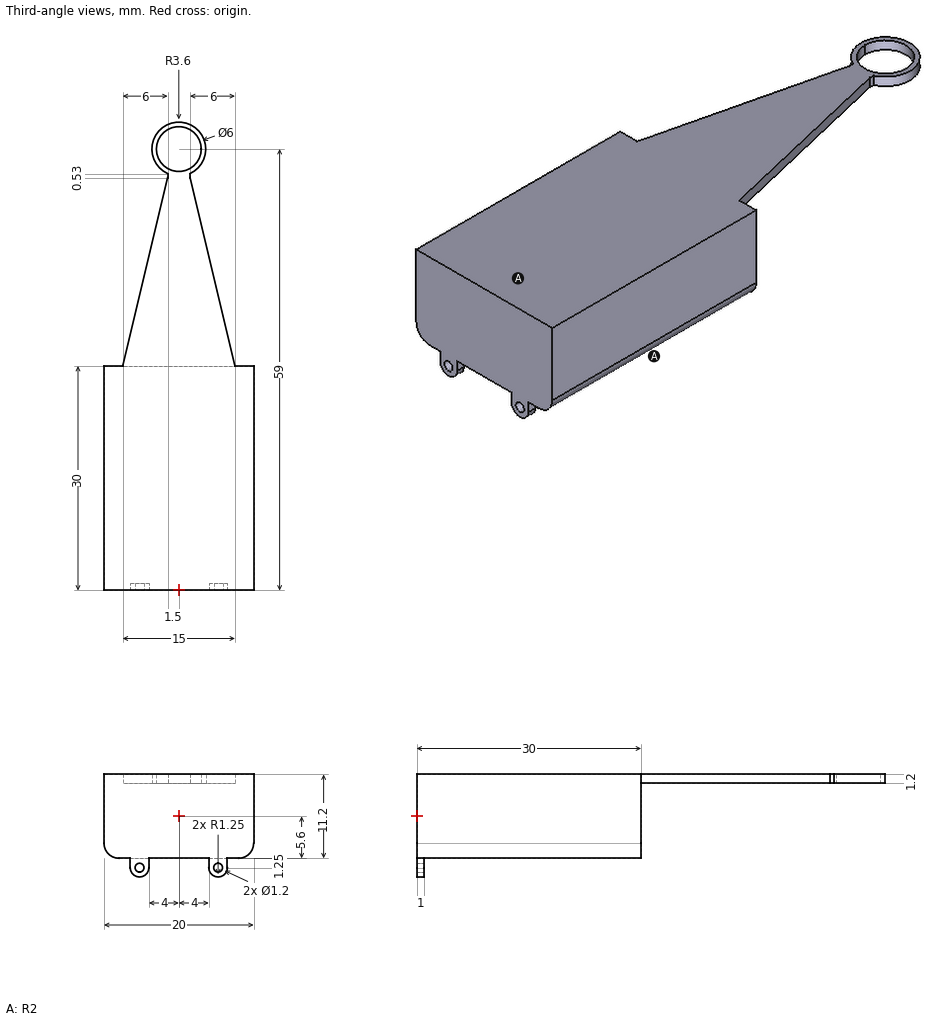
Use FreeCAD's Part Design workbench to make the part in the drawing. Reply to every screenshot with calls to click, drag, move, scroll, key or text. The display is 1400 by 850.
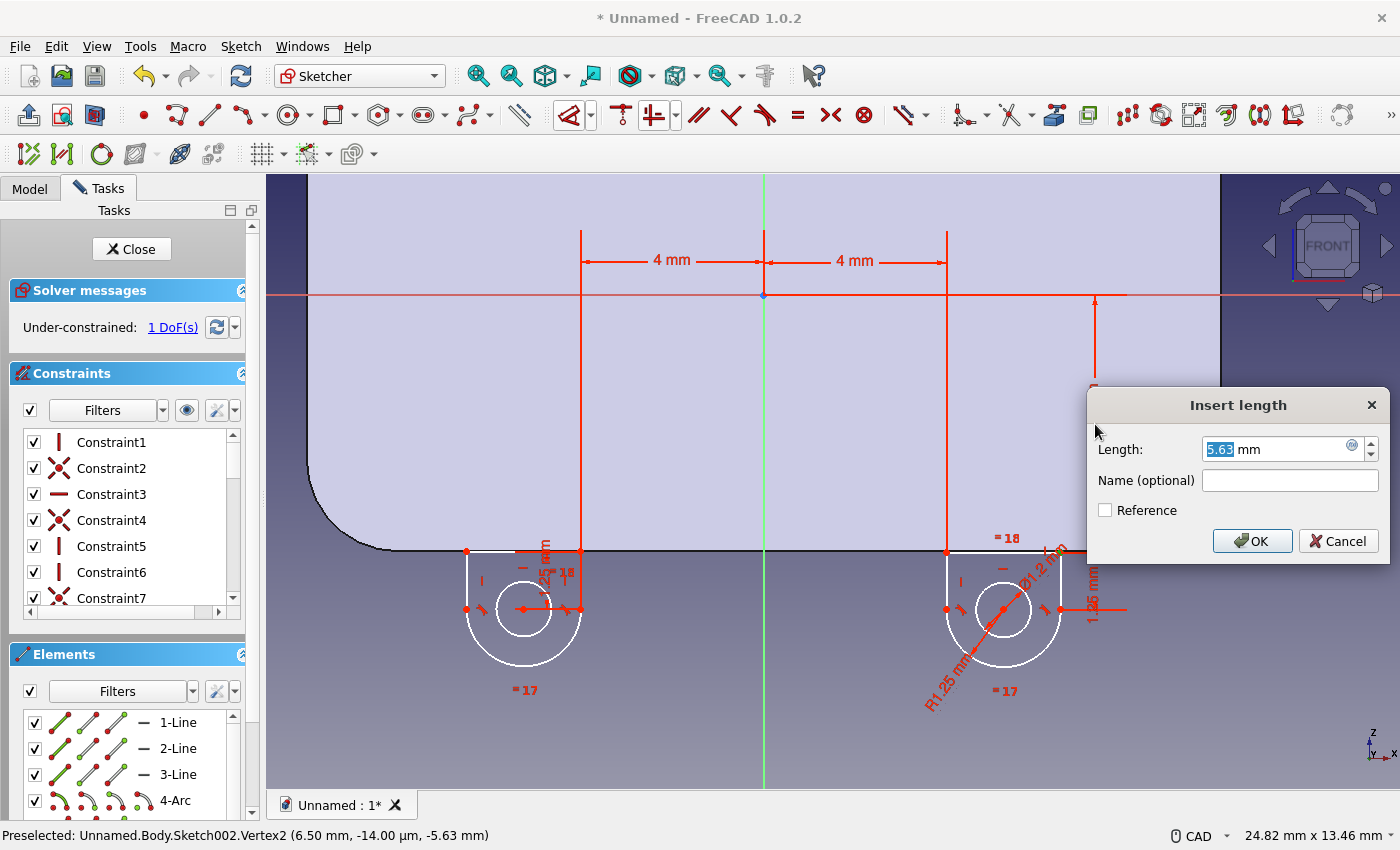
text(5.6)
key(Return)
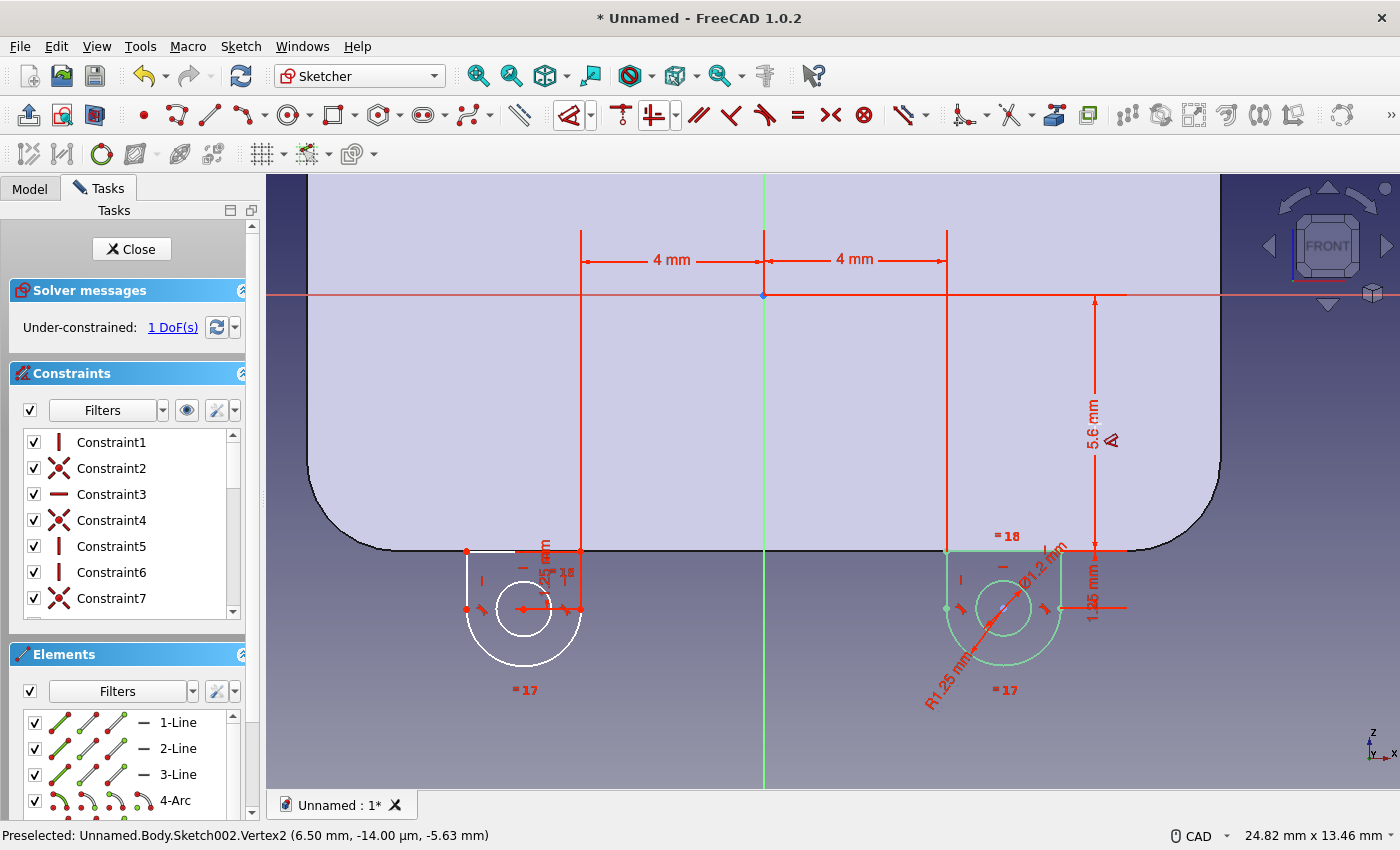
click(581, 552)
click(547, 424)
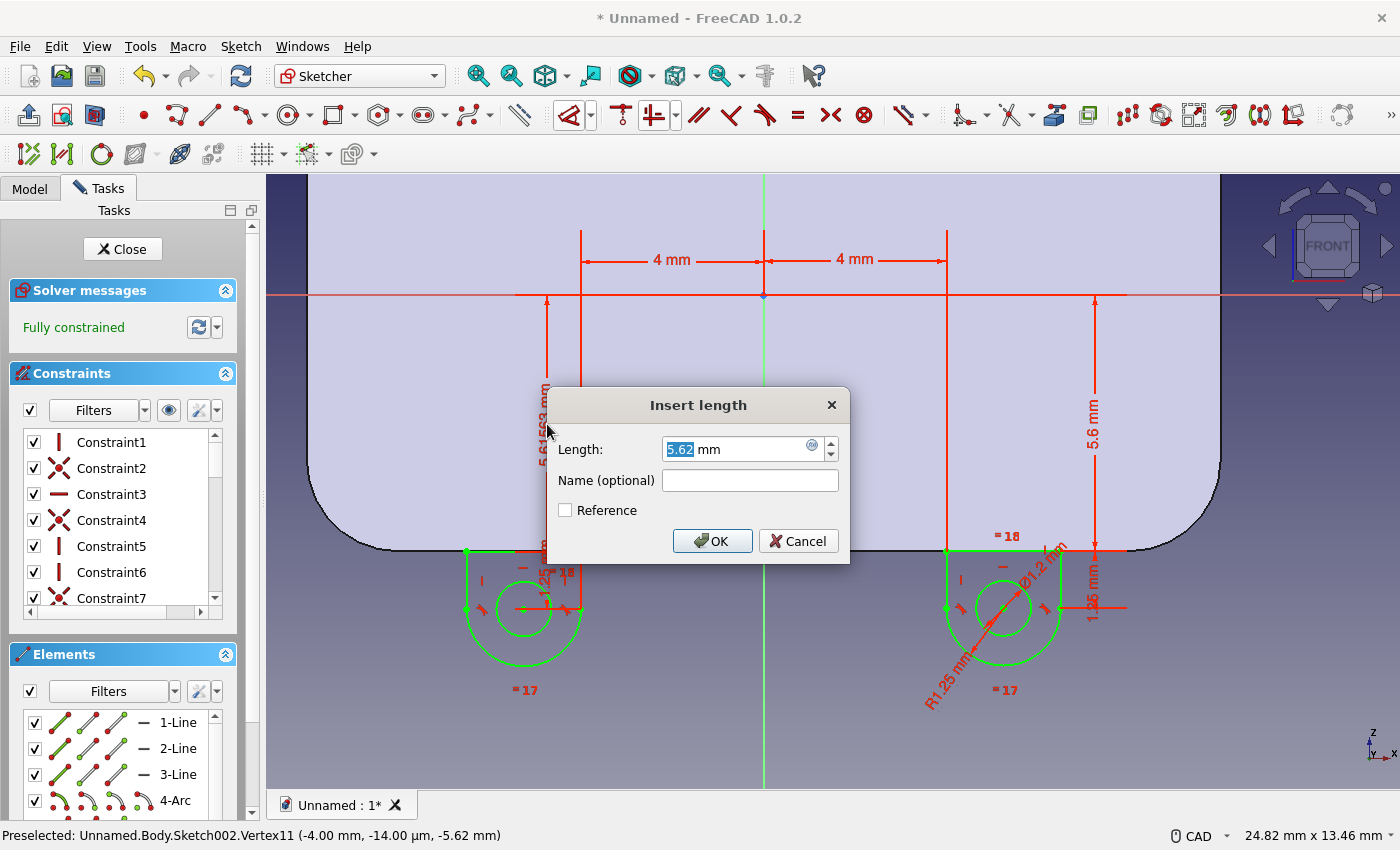
text(5.6)
key(Return)
key(Escape)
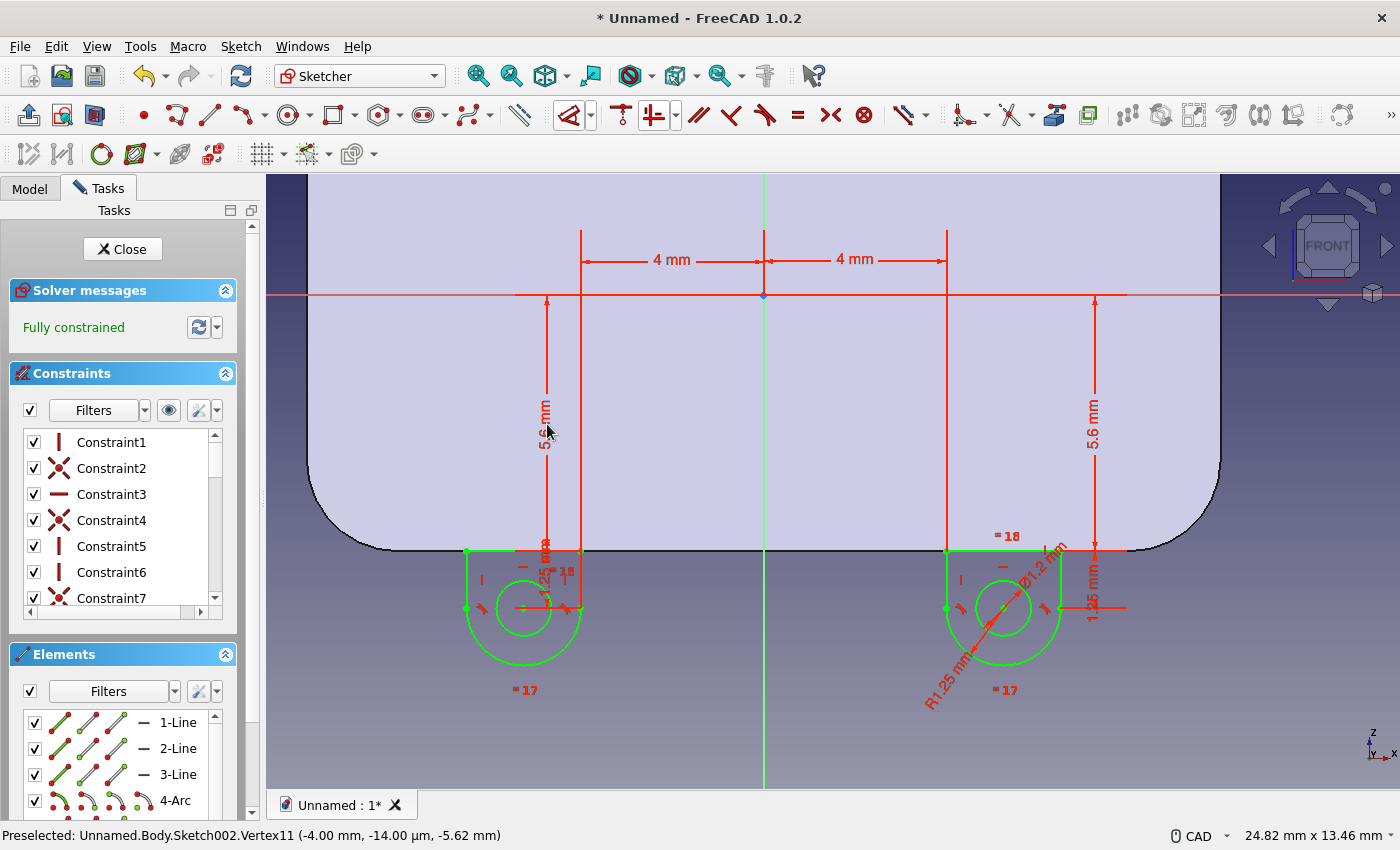
click(123, 249)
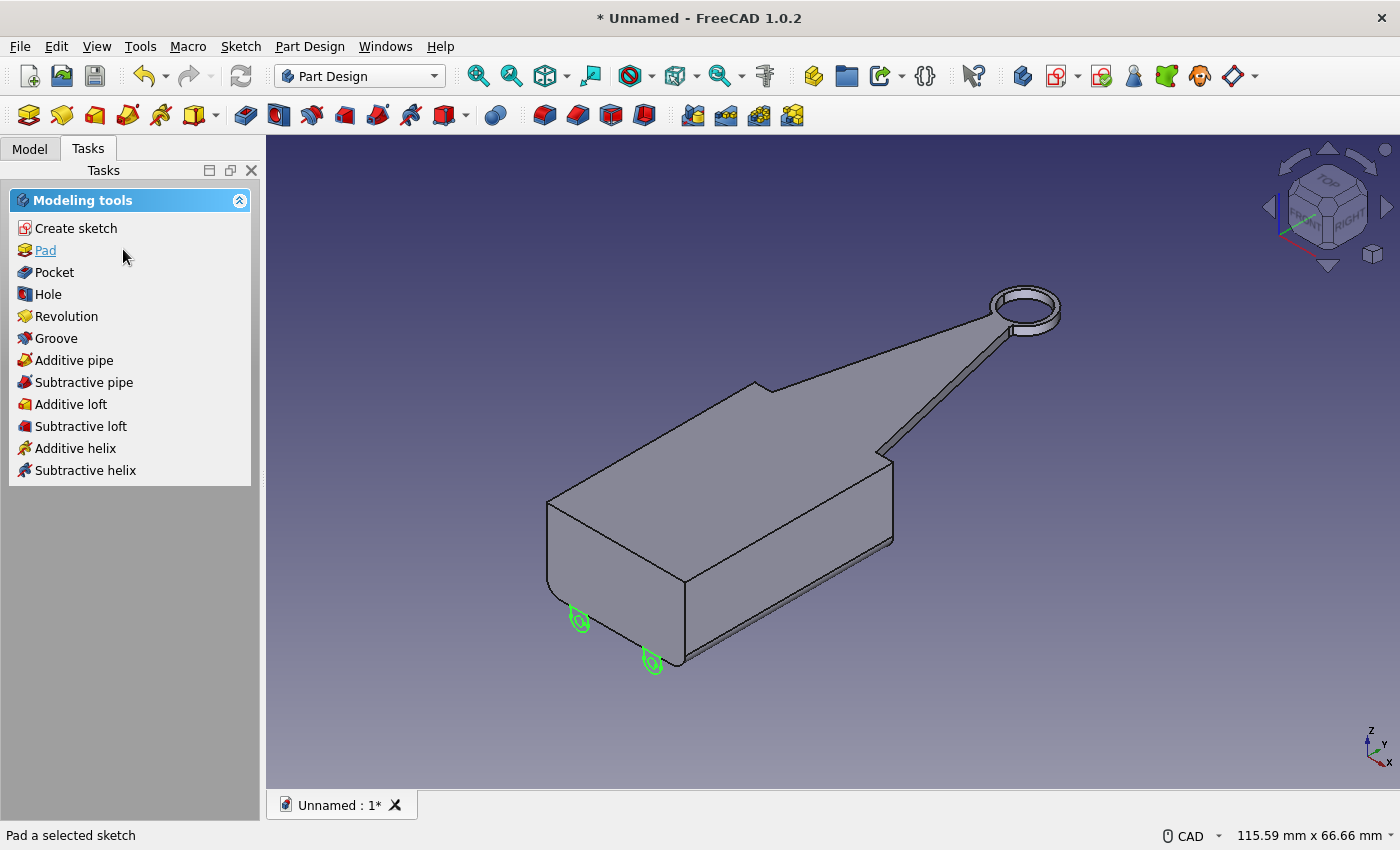
click(29, 116)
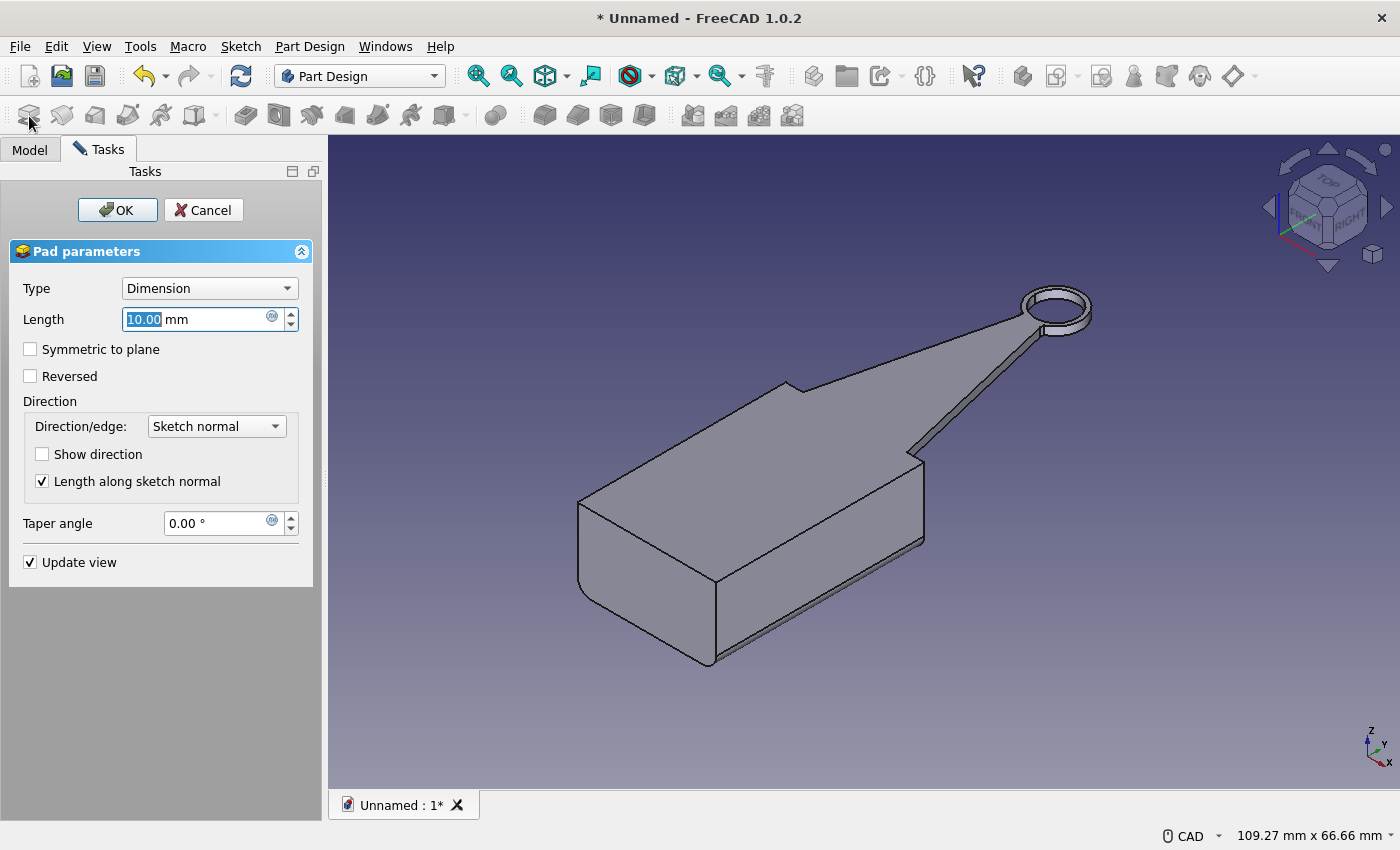
text(1)
key(Tab)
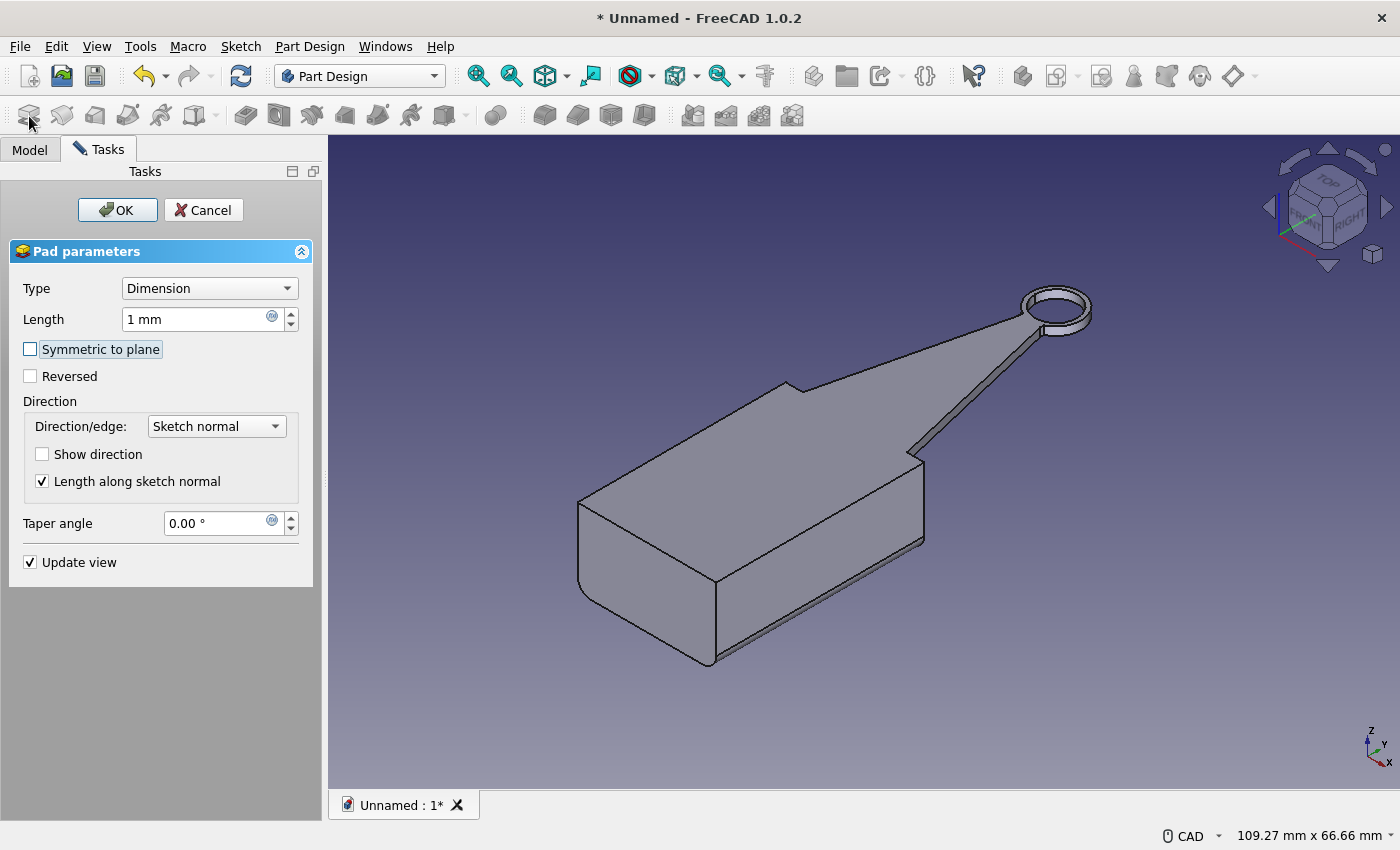
click(31, 376)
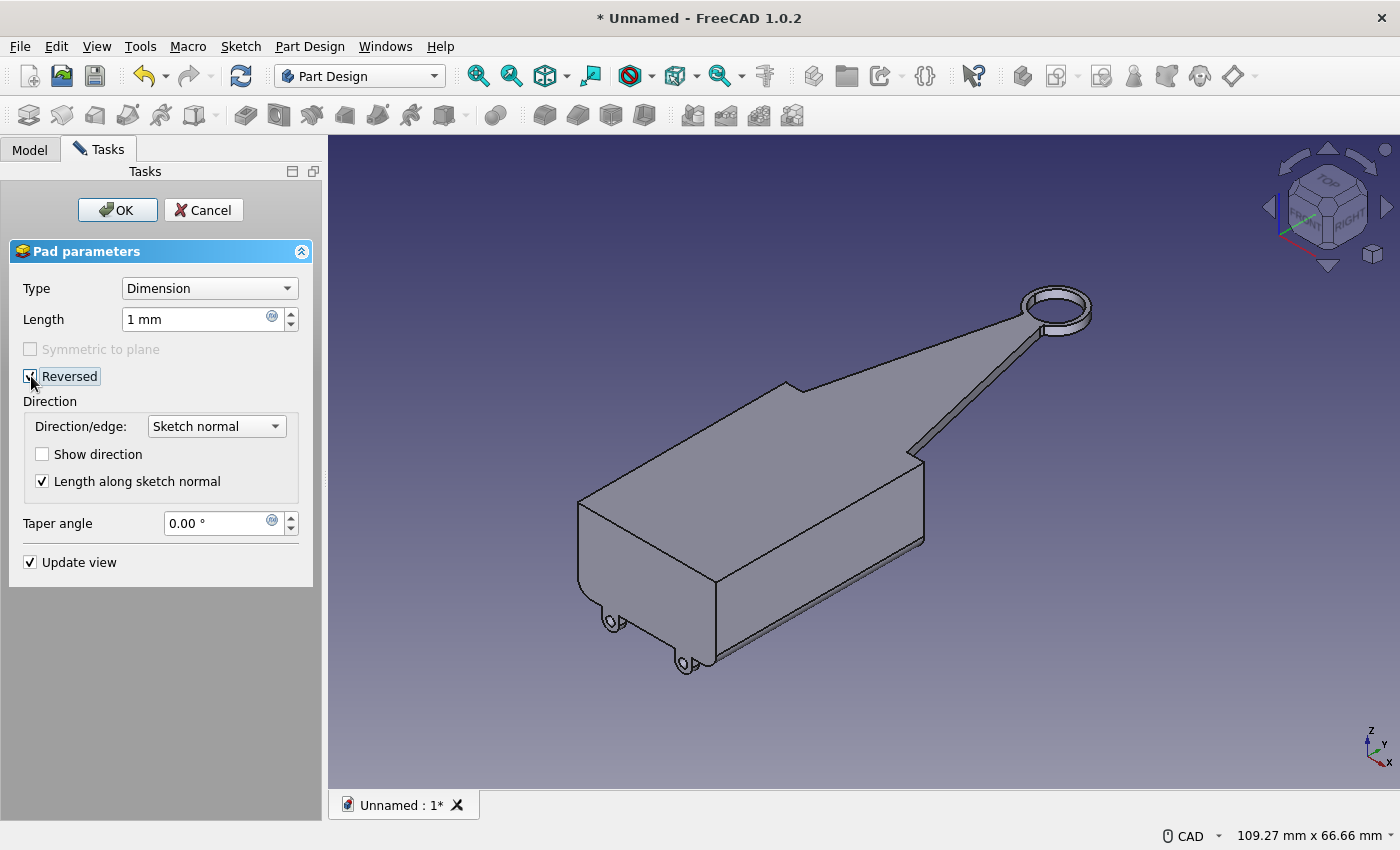
click(118, 210)